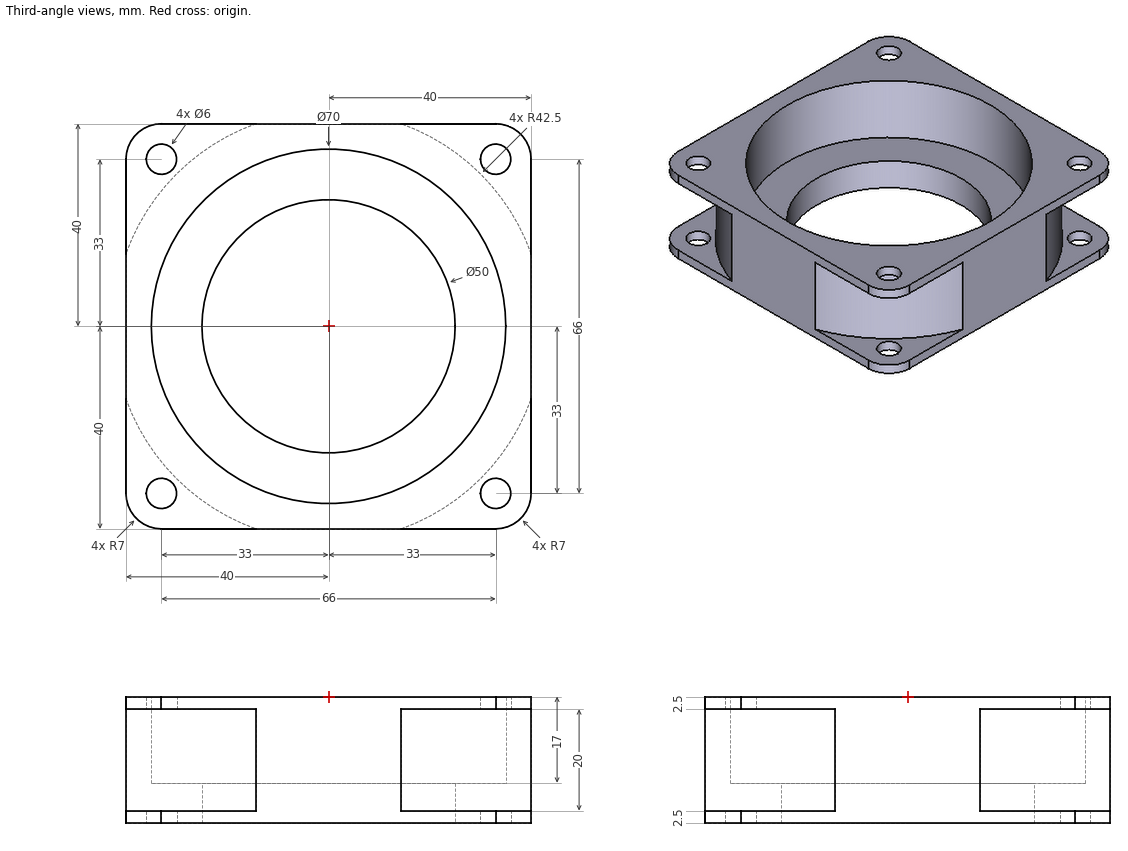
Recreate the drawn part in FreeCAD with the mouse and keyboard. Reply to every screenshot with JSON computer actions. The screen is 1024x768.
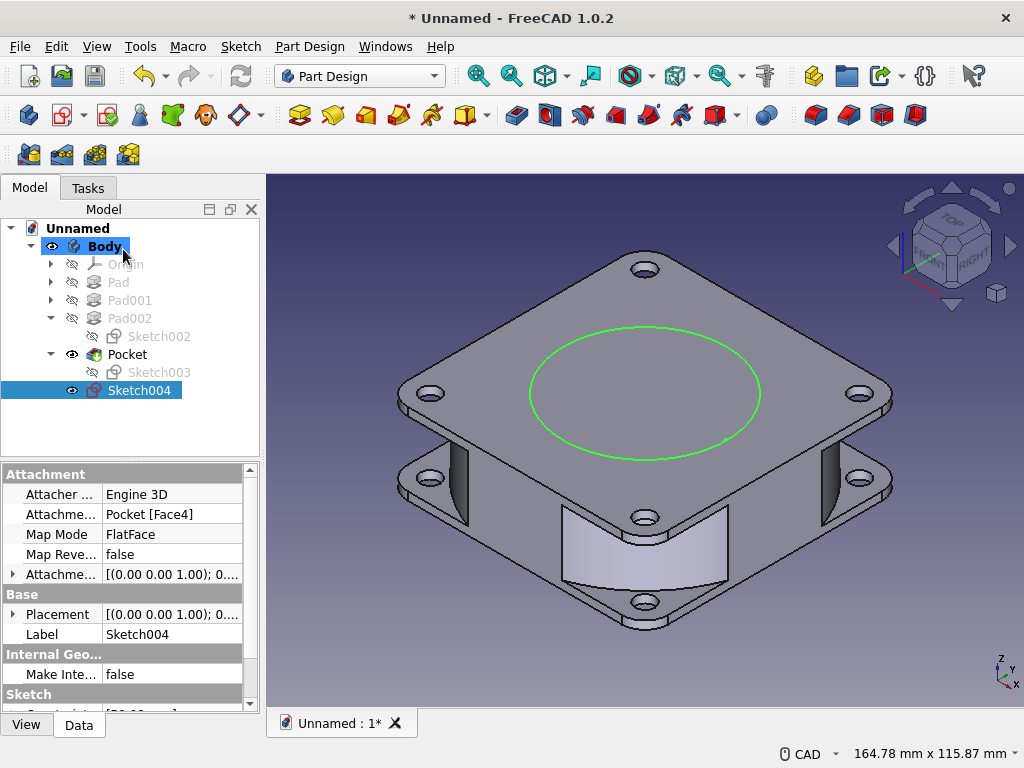
{"action": "left_click", "coordinate": [517, 116]}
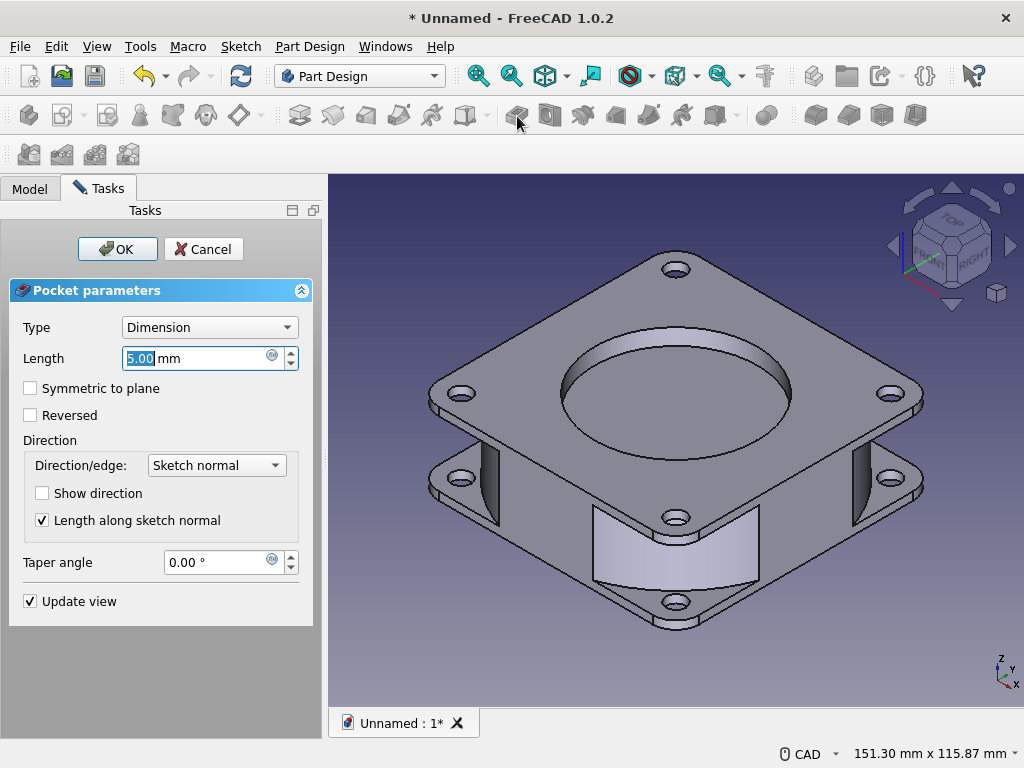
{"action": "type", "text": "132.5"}
{"action": "key", "text": "Tab"}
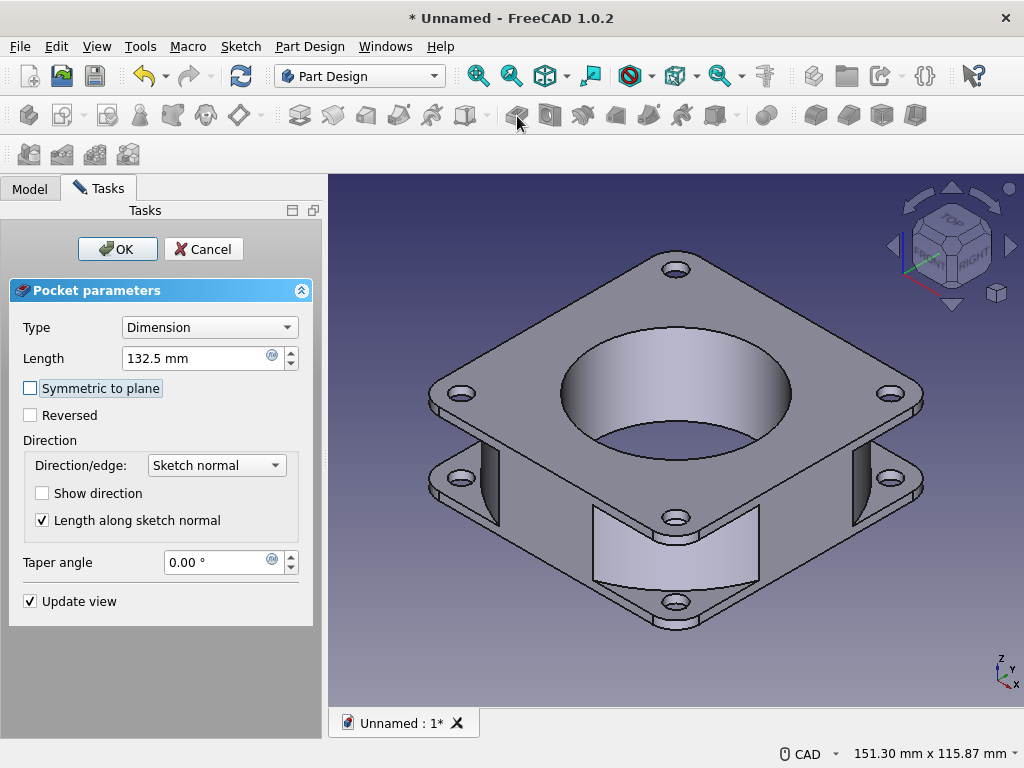
{"action": "left_click", "coordinate": [118, 249]}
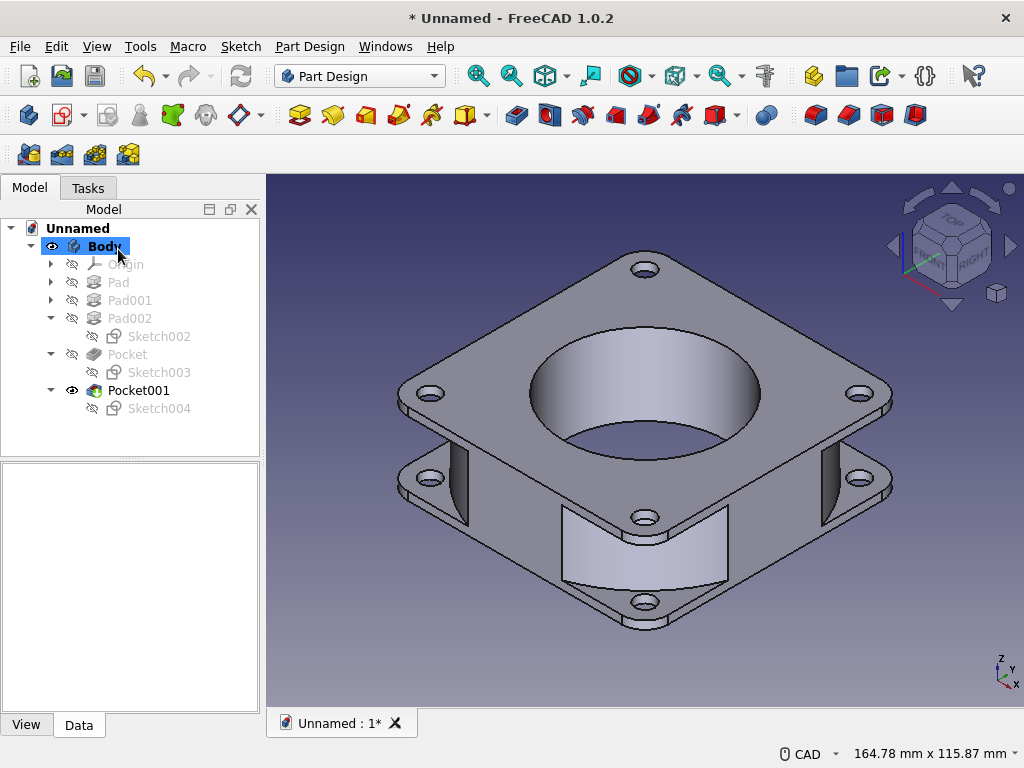
{"action": "left_click", "coordinate": [645, 478]}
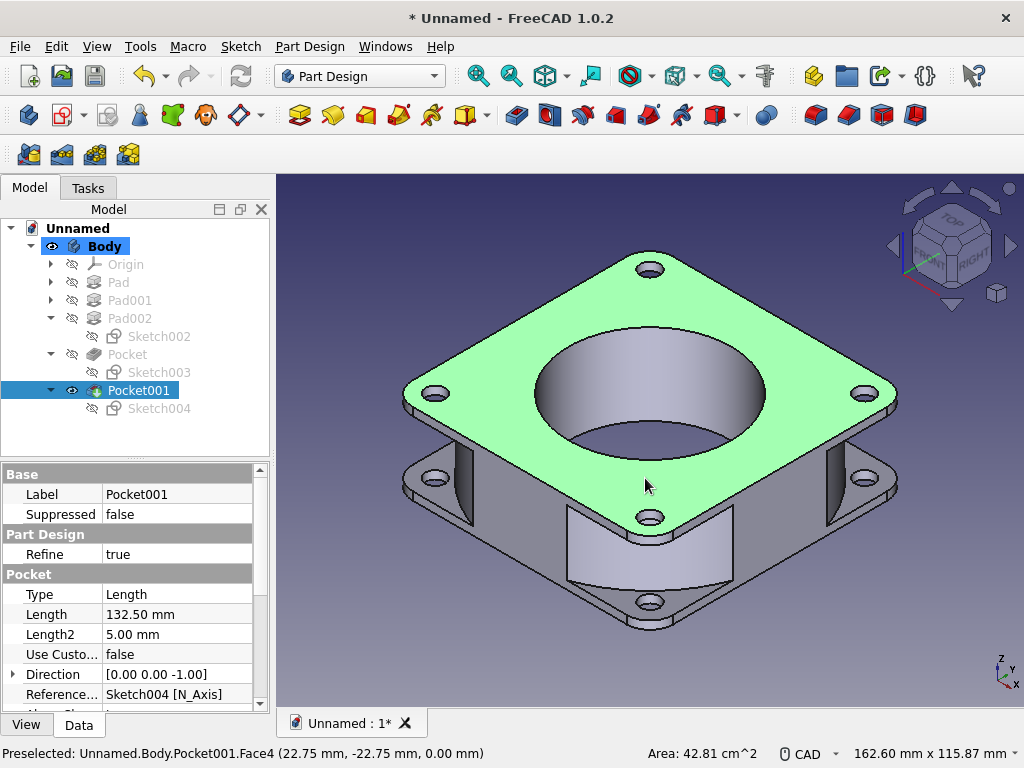
{"action": "left_click", "coordinate": [62, 116]}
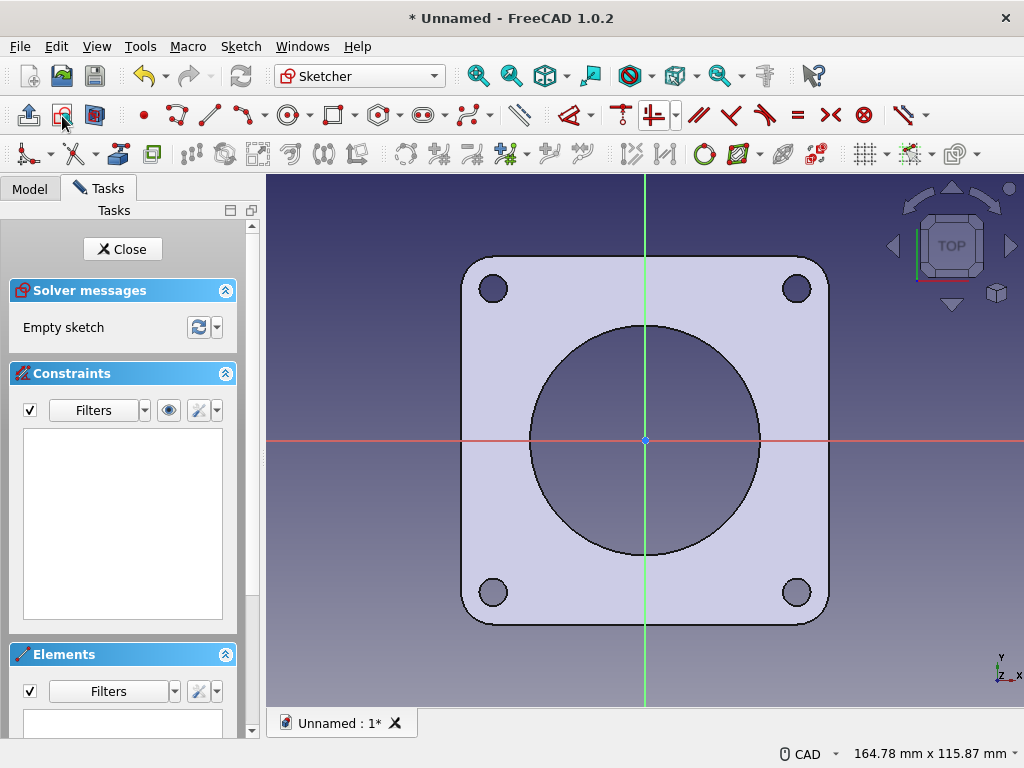
{"action": "left_click", "coordinate": [288, 116]}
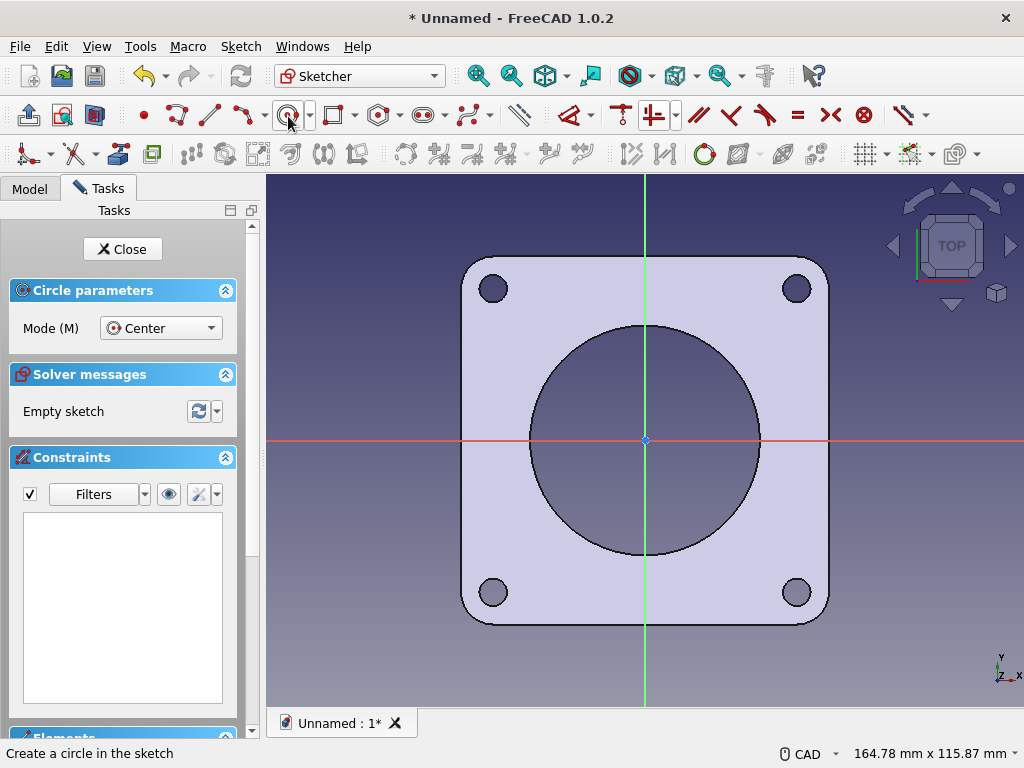
{"action": "left_click", "coordinate": [645, 440]}
{"action": "mouse_move", "coordinate": [759, 327]}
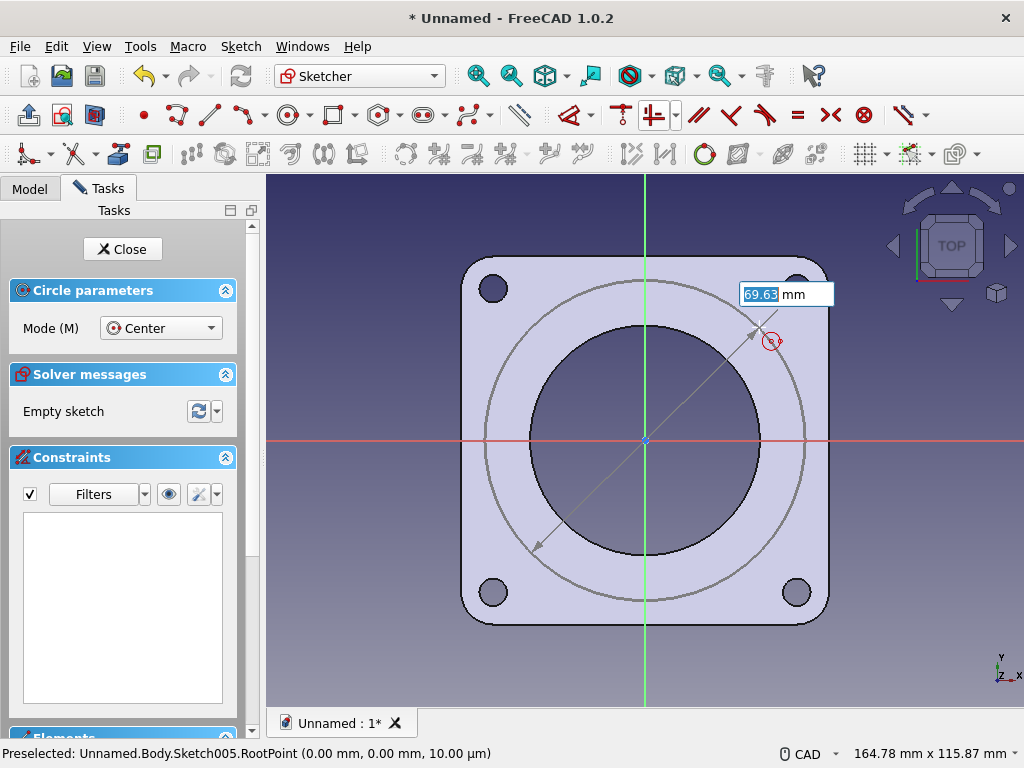
{"action": "type", "text": "70"}
{"action": "key", "text": "Return"}
{"action": "key", "text": "Escape"}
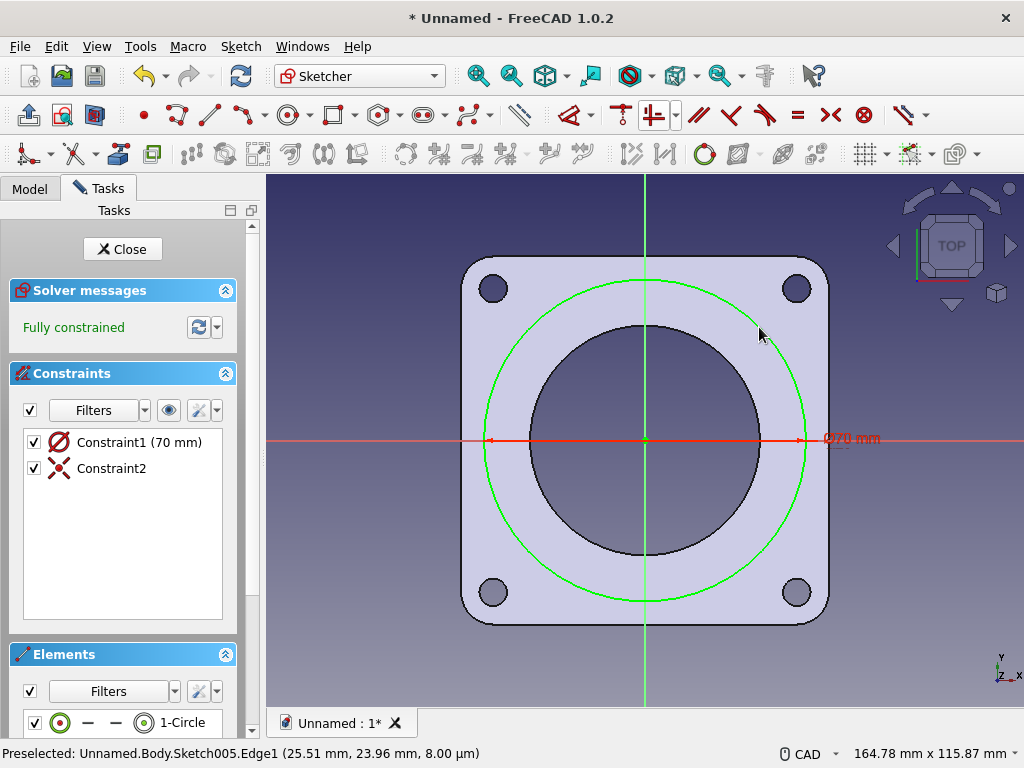
{"action": "left_click", "coordinate": [123, 249]}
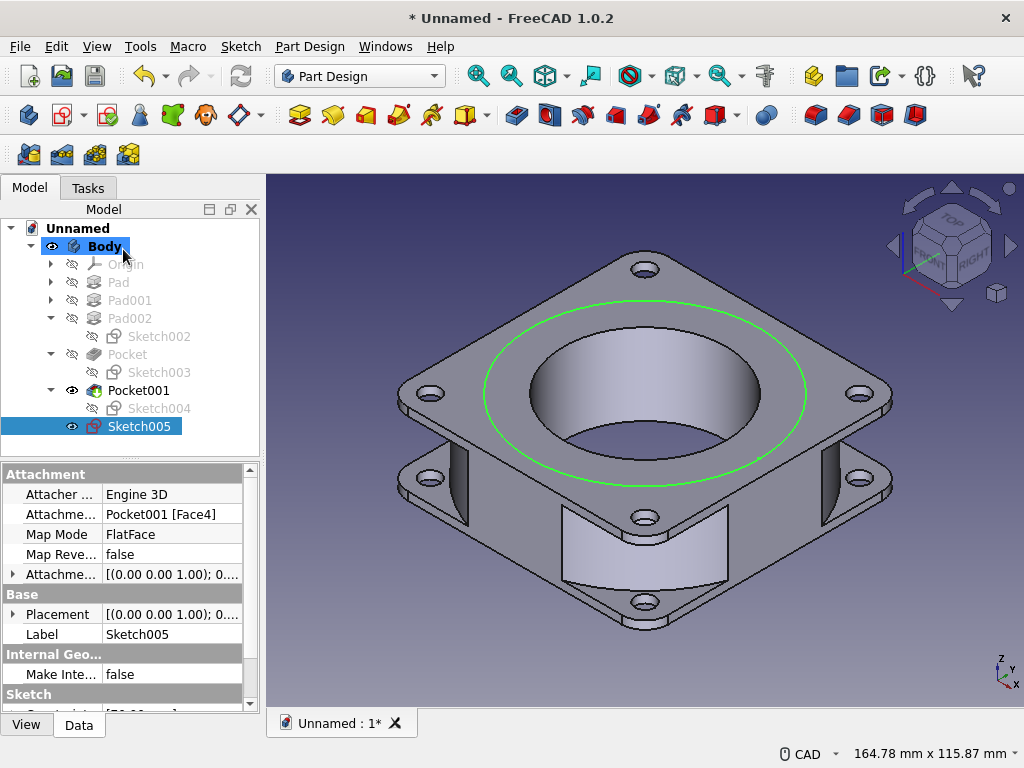
{"action": "left_click", "coordinate": [517, 116]}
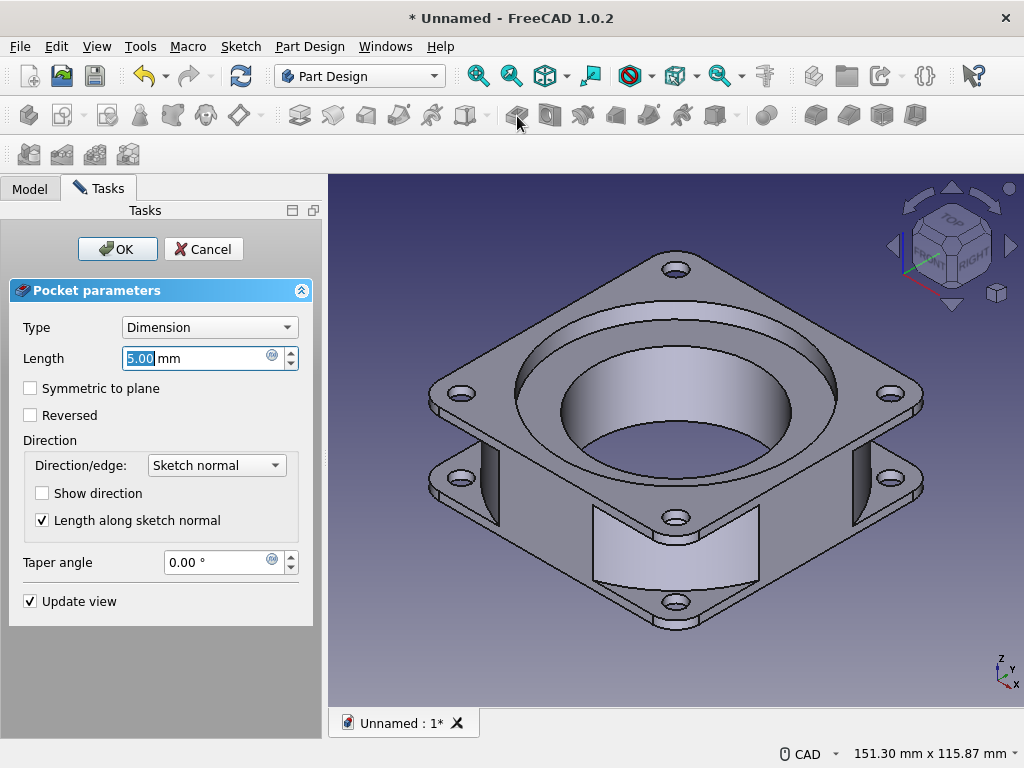
{"action": "type", "text": "17"}
{"action": "key", "text": "Tab"}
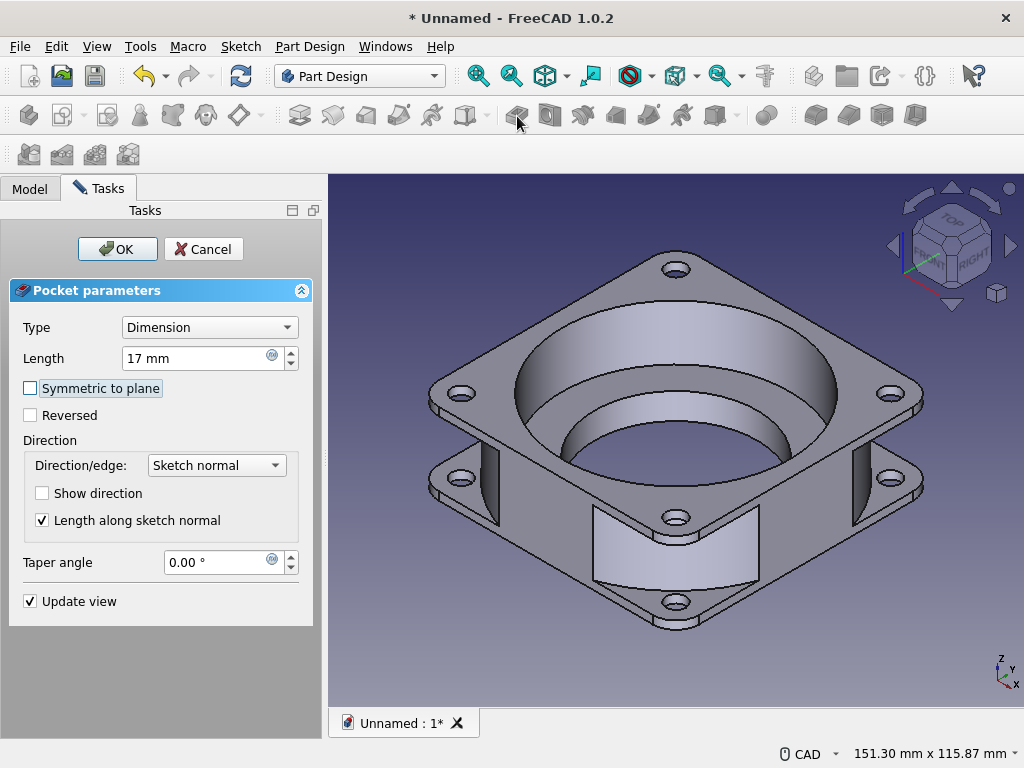
{"action": "left_click", "coordinate": [118, 249]}